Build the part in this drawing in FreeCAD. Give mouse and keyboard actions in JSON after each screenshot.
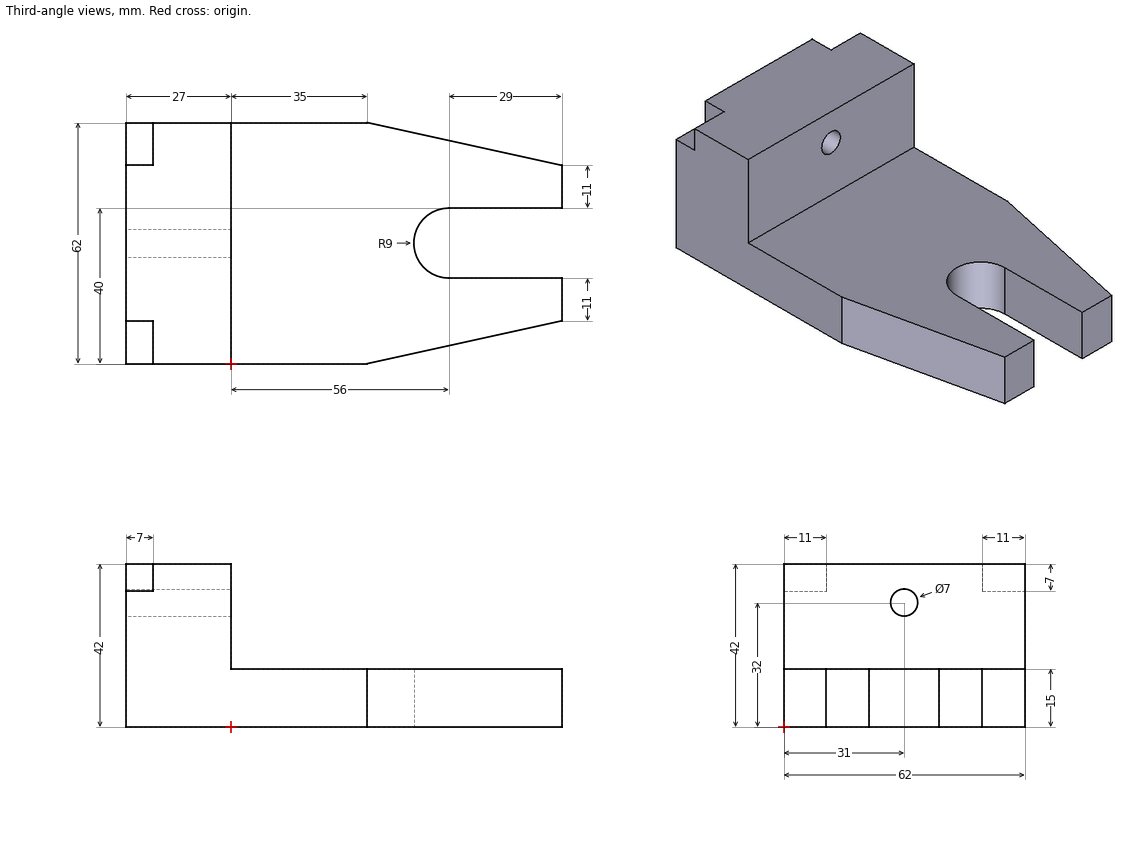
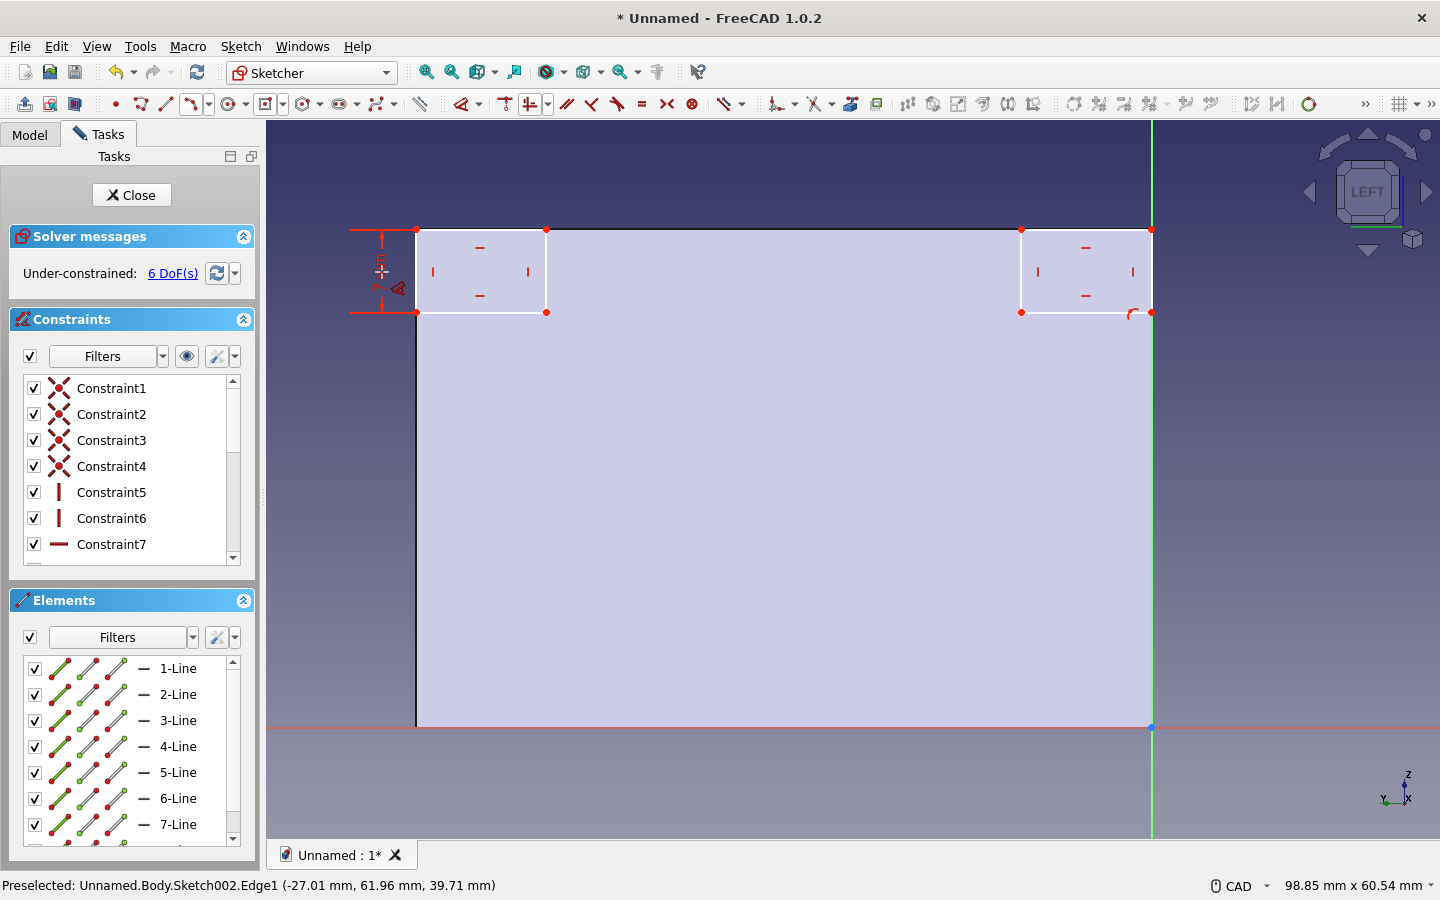
{"action": "left_click", "coordinate": [1021, 255]}
{"action": "left_click", "coordinate": [1055, 272]}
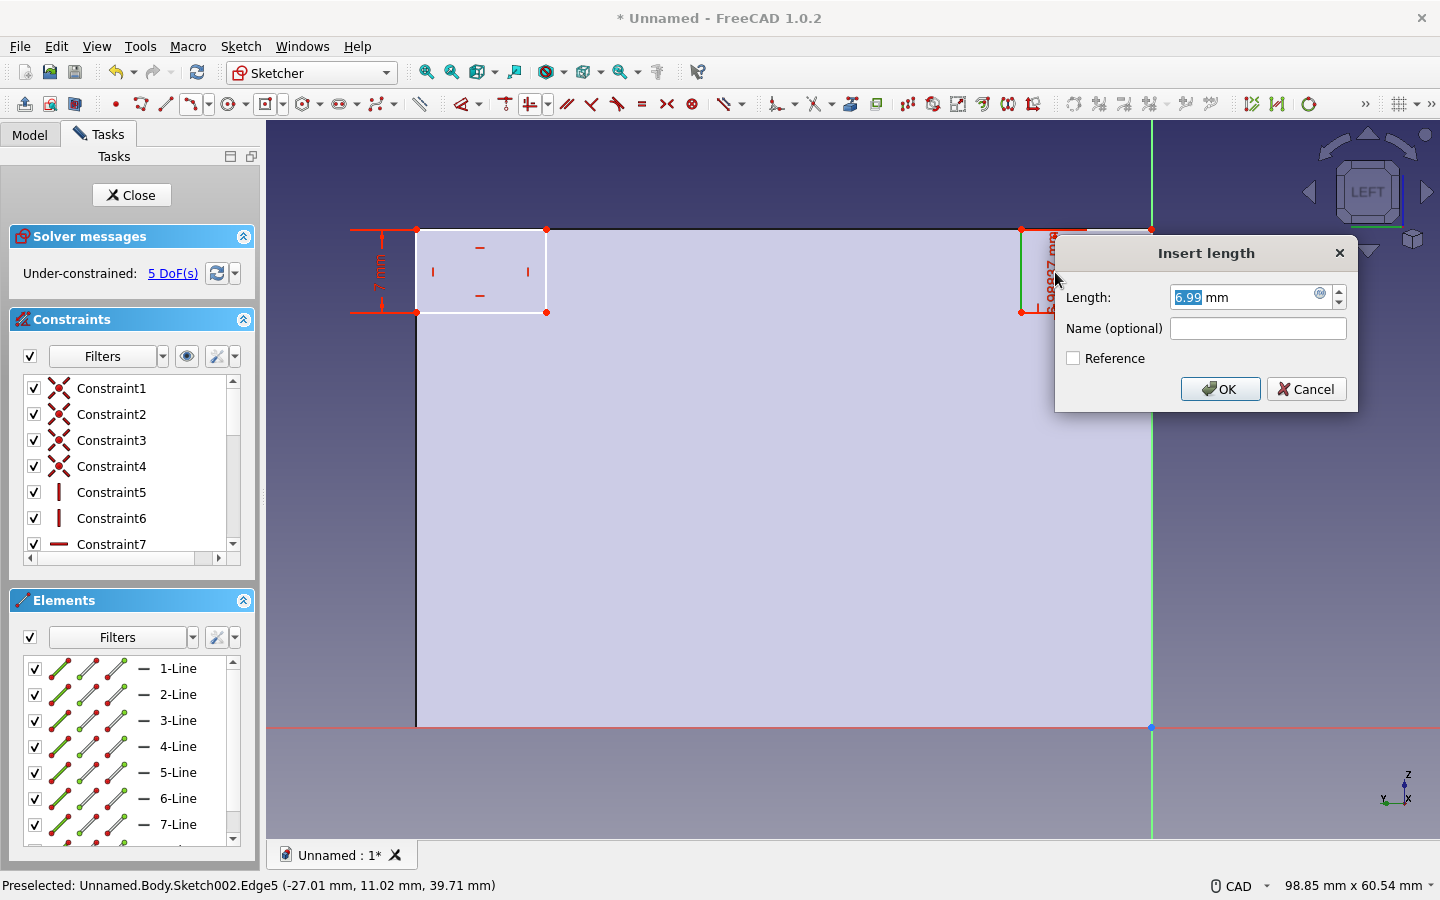
{"action": "type", "text": "7"}
{"action": "key", "text": "Return"}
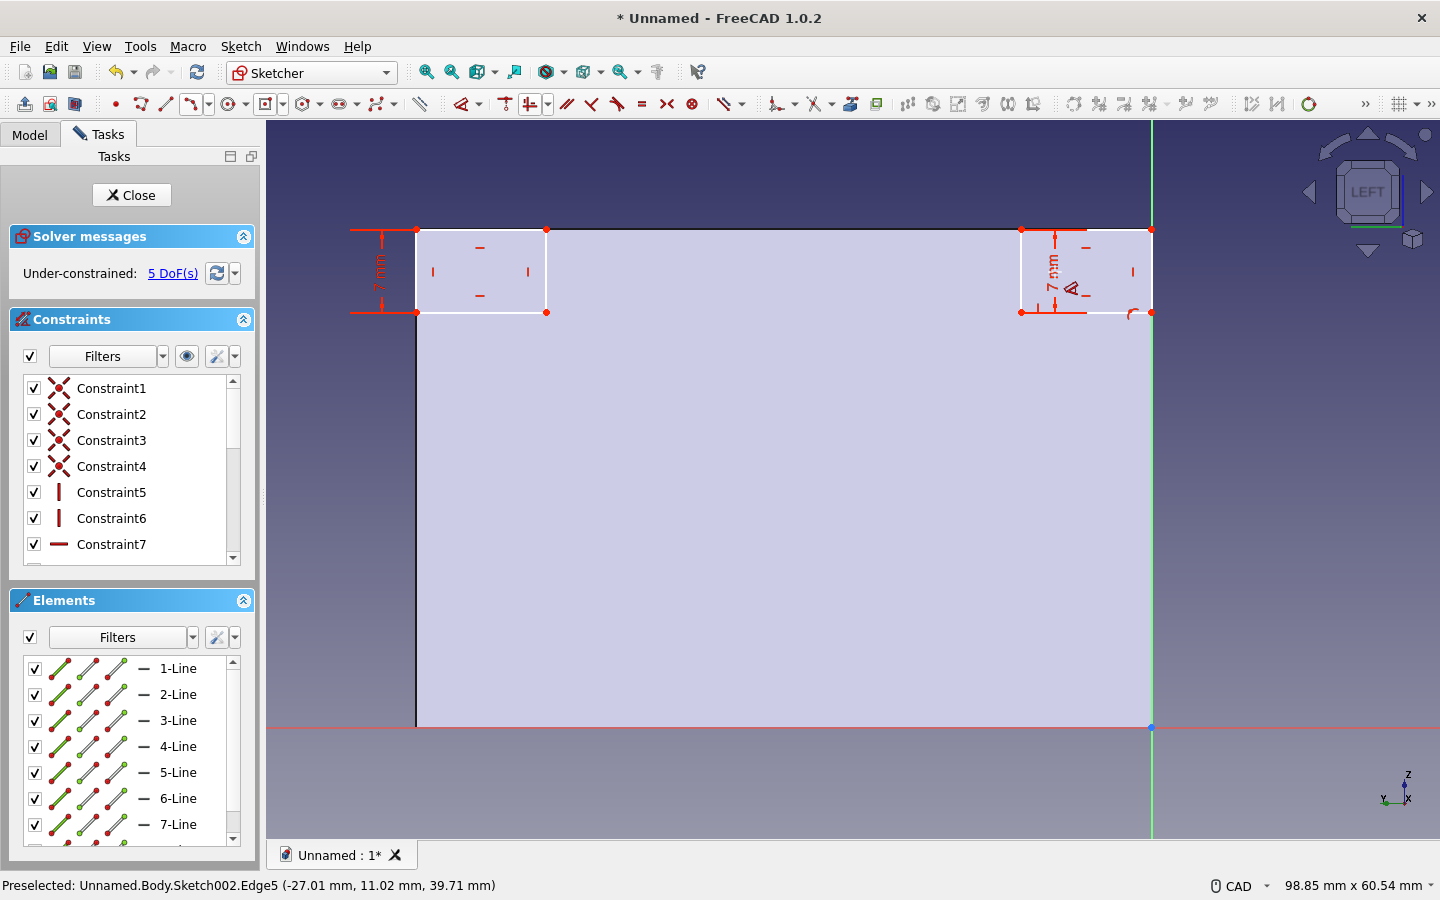
{"action": "left_click", "coordinate": [455, 313]}
{"action": "left_click", "coordinate": [481, 279]}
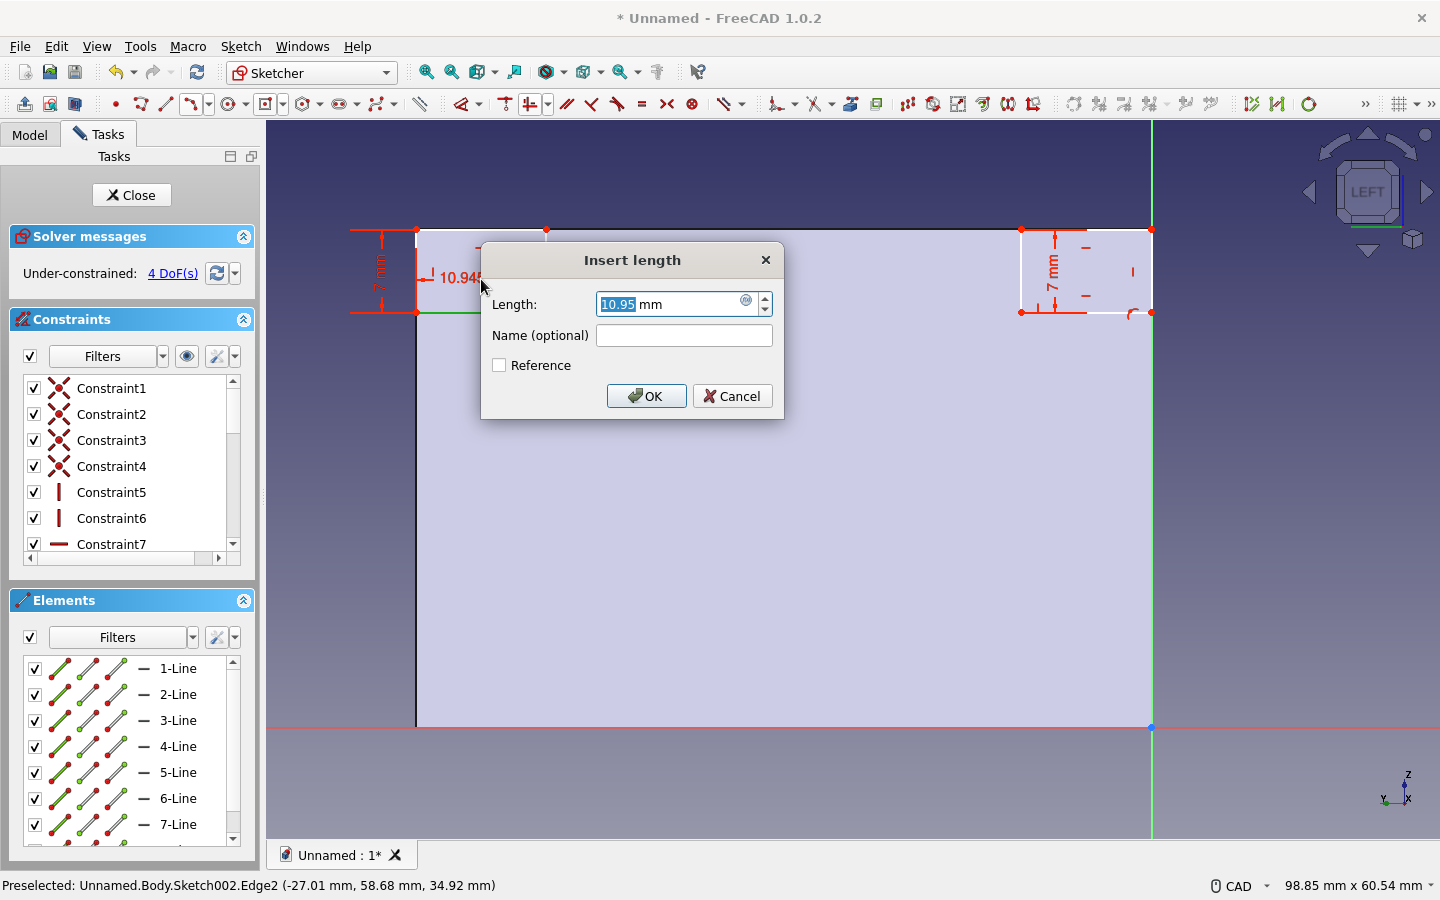
{"action": "type", "text": "11"}
{"action": "key", "text": "Return"}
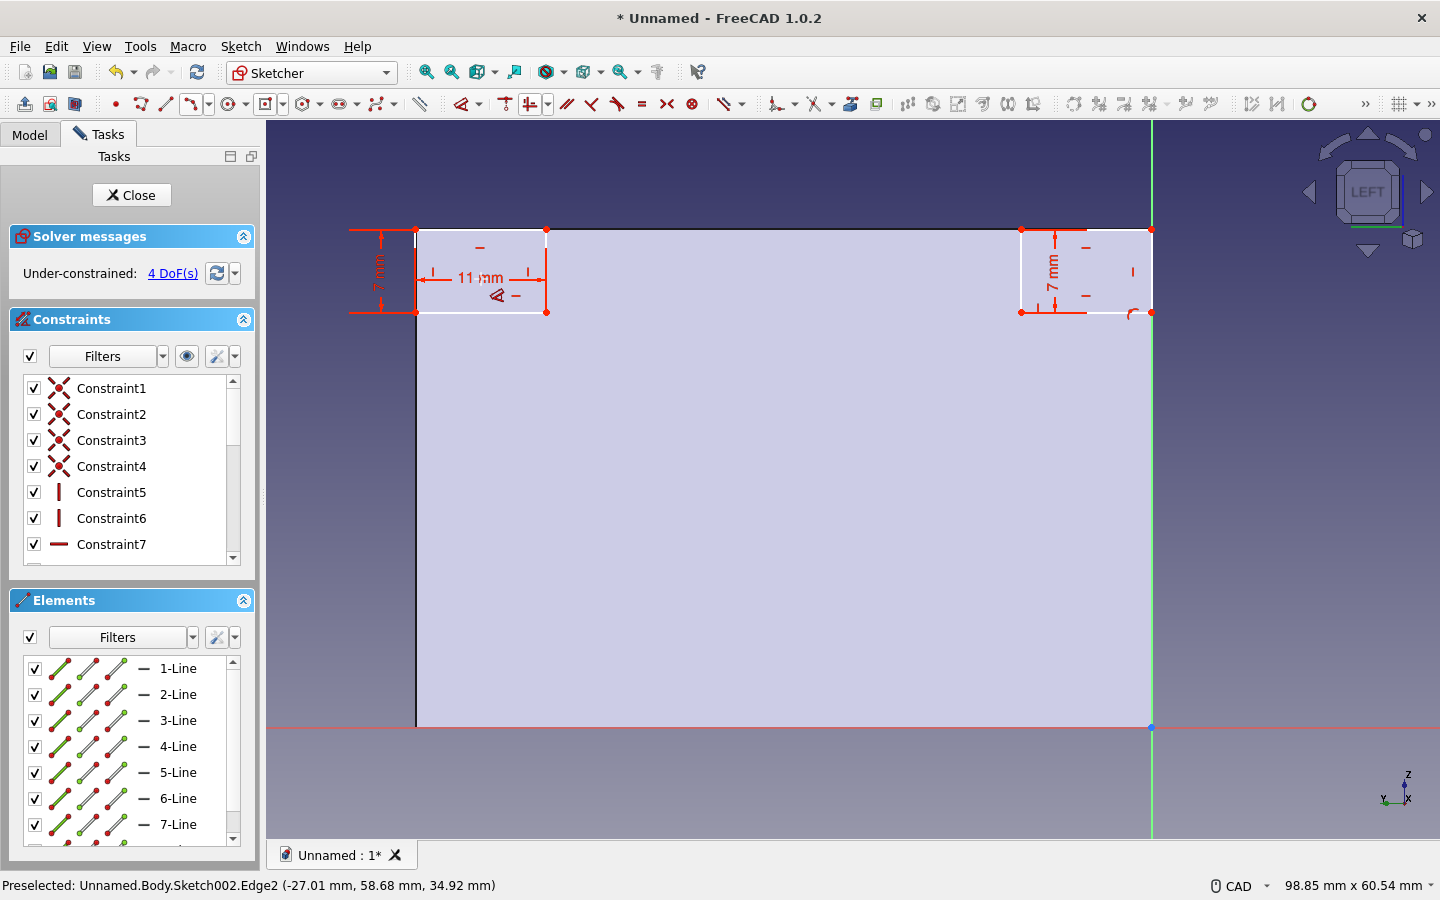
{"action": "left_click", "coordinate": [1060, 313]}
{"action": "left_click", "coordinate": [1132, 279]}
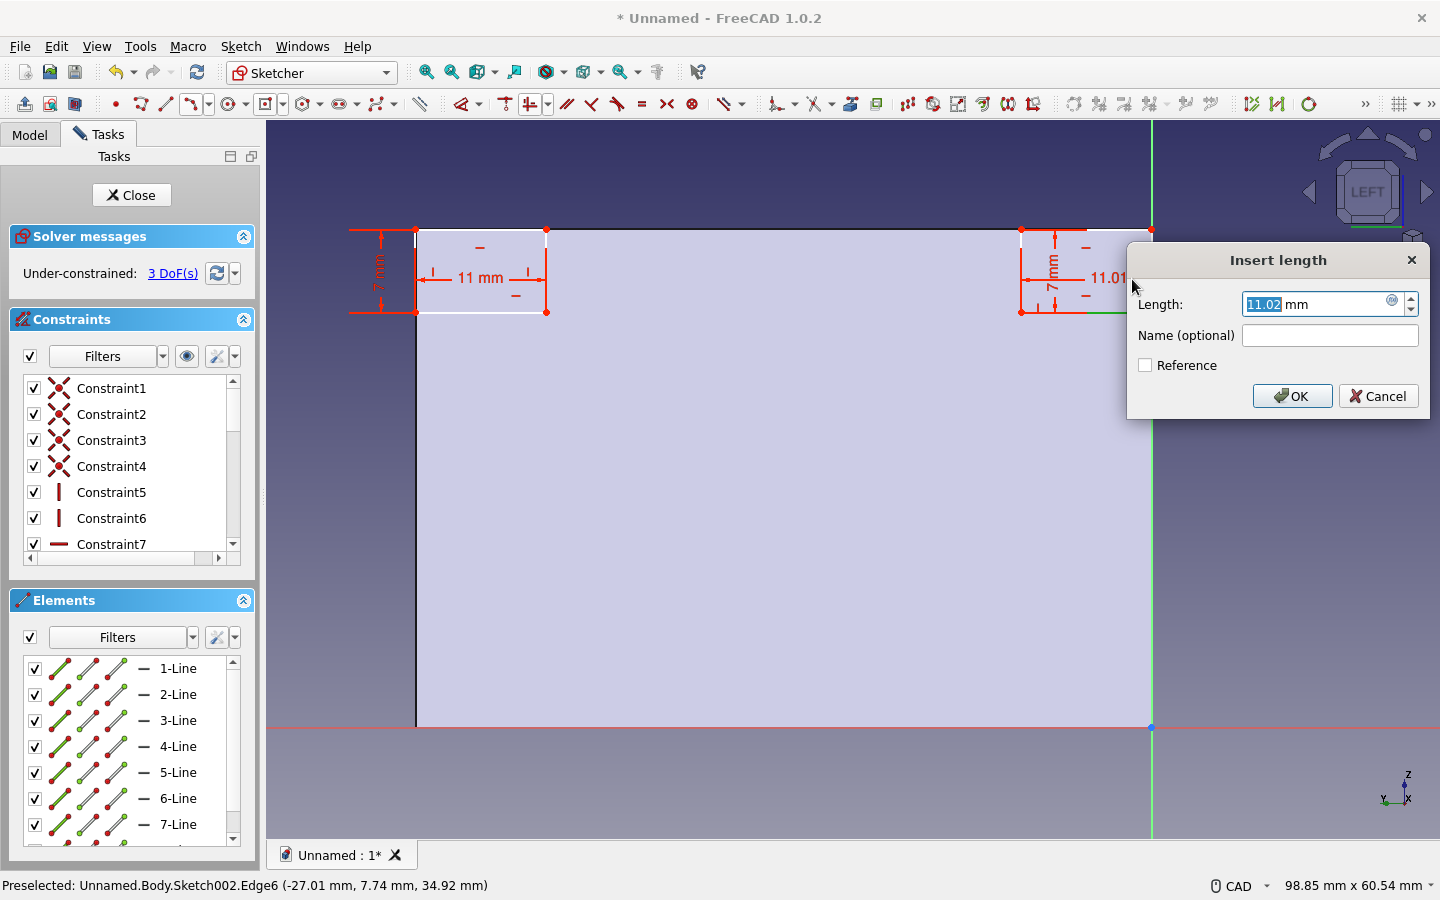
{"action": "type", "text": "11"}
{"action": "key", "text": "Return"}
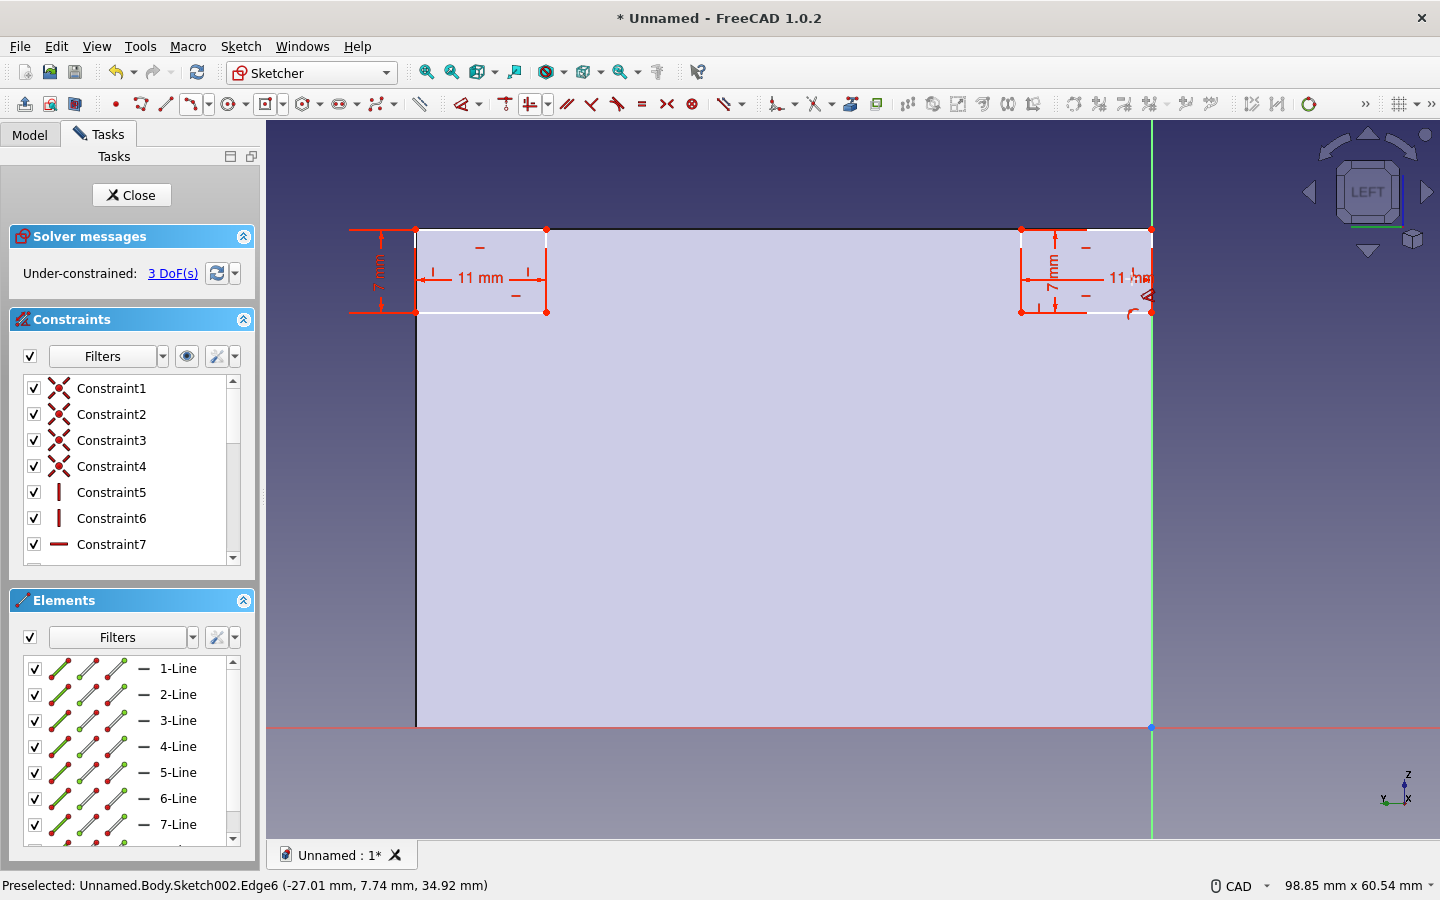
{"action": "left_click", "coordinate": [415, 230]}
{"action": "left_click", "coordinate": [784, 762]}